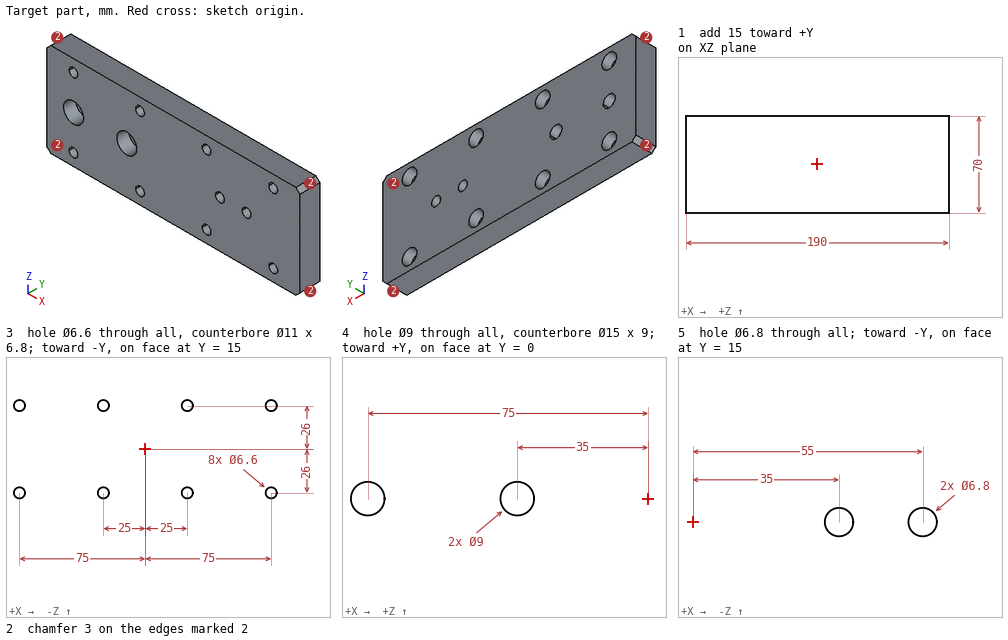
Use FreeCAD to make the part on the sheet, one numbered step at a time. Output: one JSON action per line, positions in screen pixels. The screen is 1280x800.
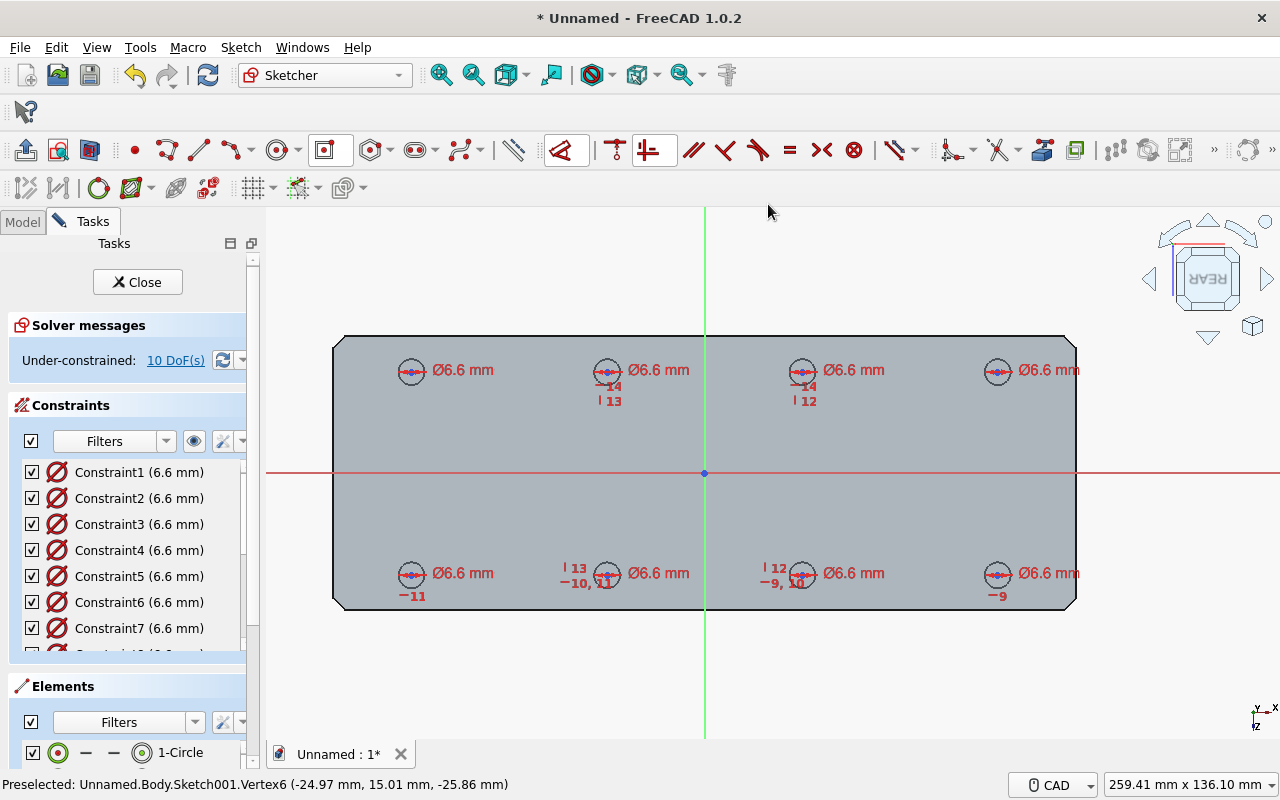
{"action": "left_click", "coordinate": [412, 575]}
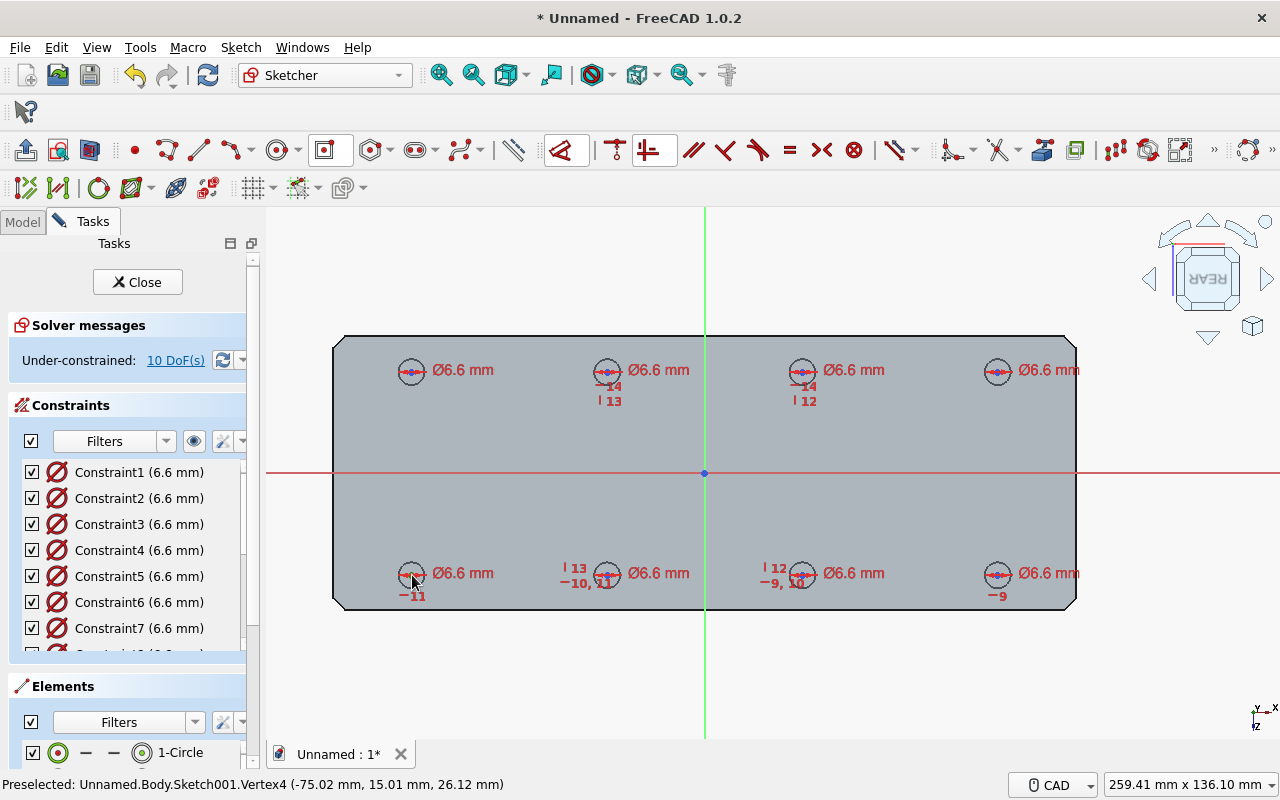
{"action": "left_click", "coordinate": [412, 372]}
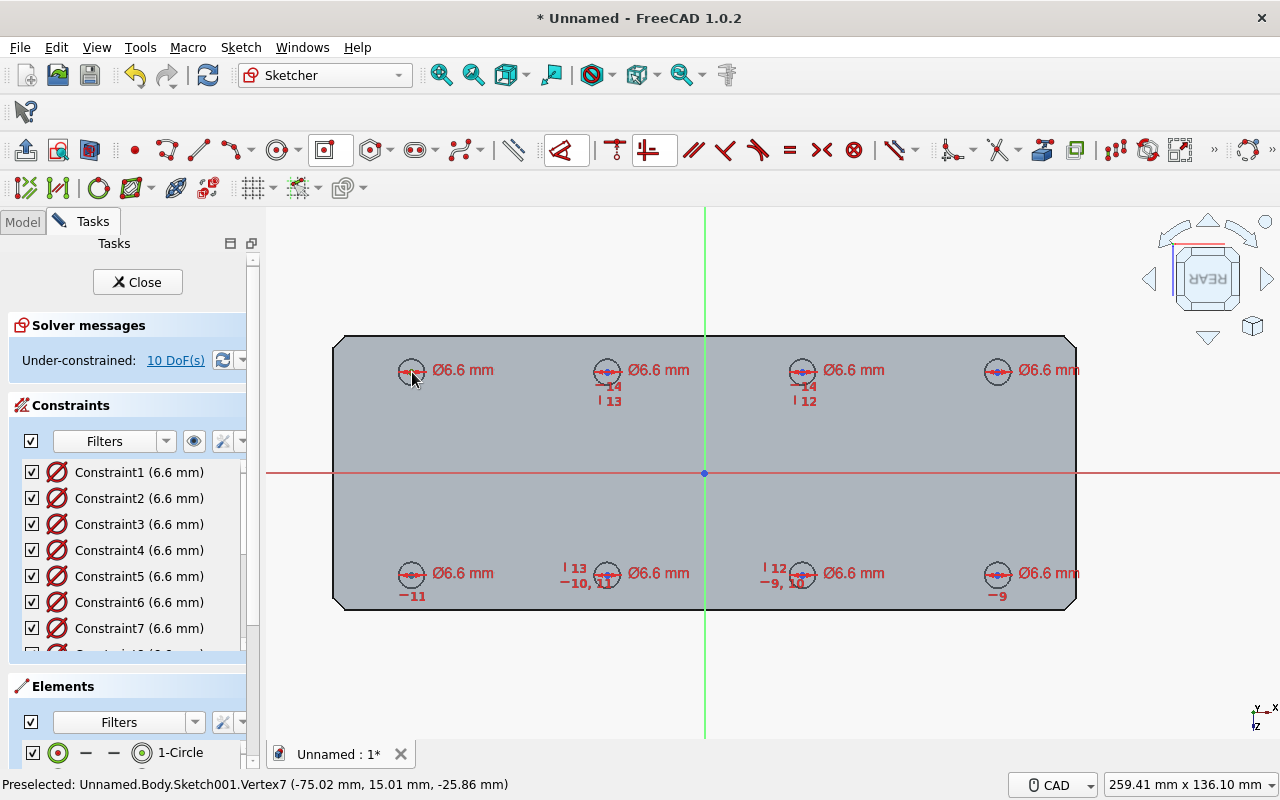
{"action": "key", "text": "v"}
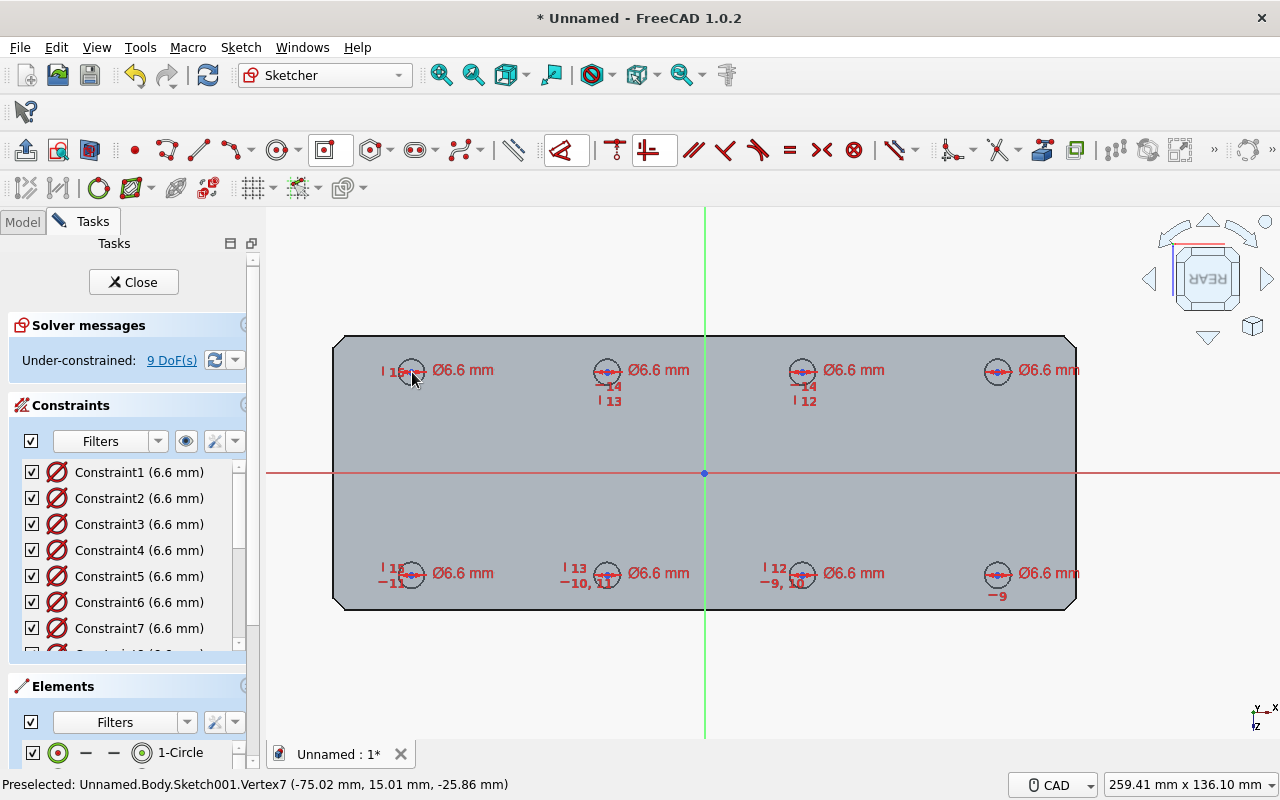
{"action": "left_click", "coordinate": [607, 372]}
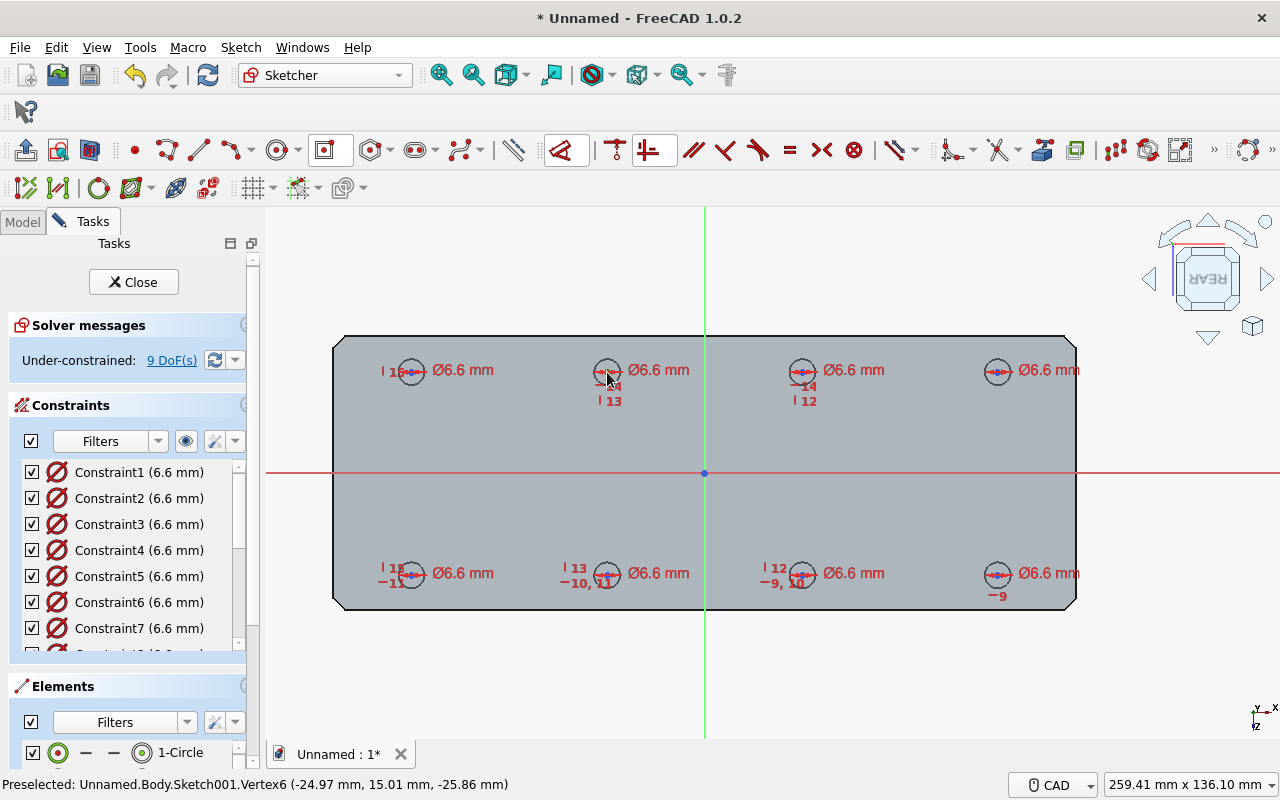
{"action": "left_click", "coordinate": [412, 372]}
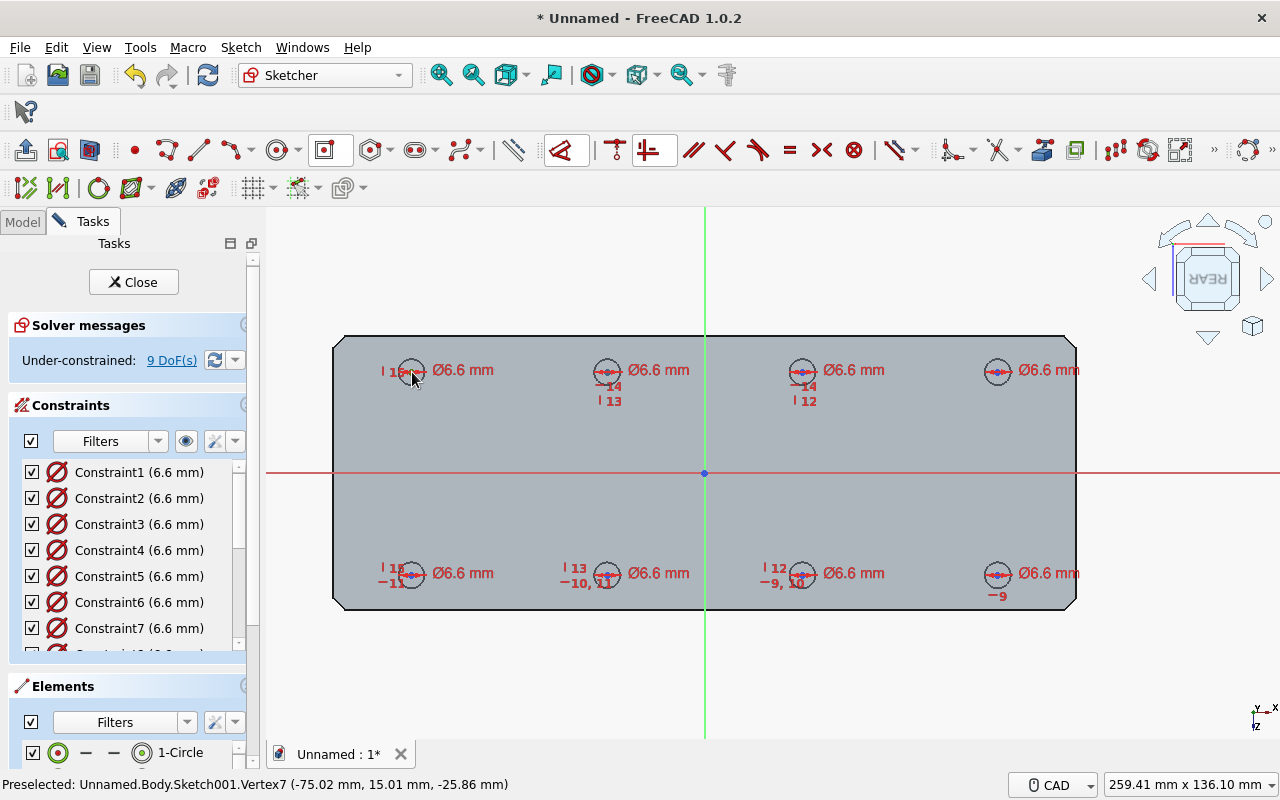
{"action": "key", "text": "h"}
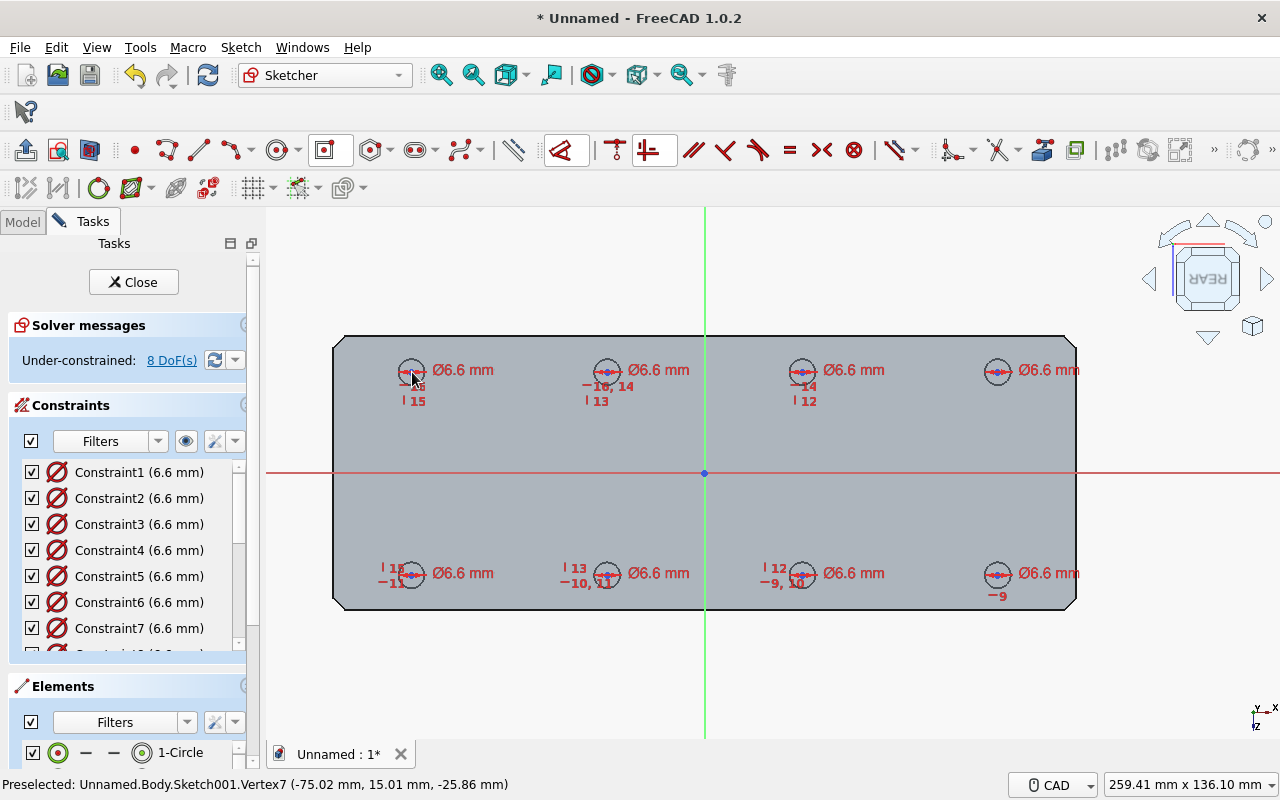
{"action": "left_click", "coordinate": [998, 575]}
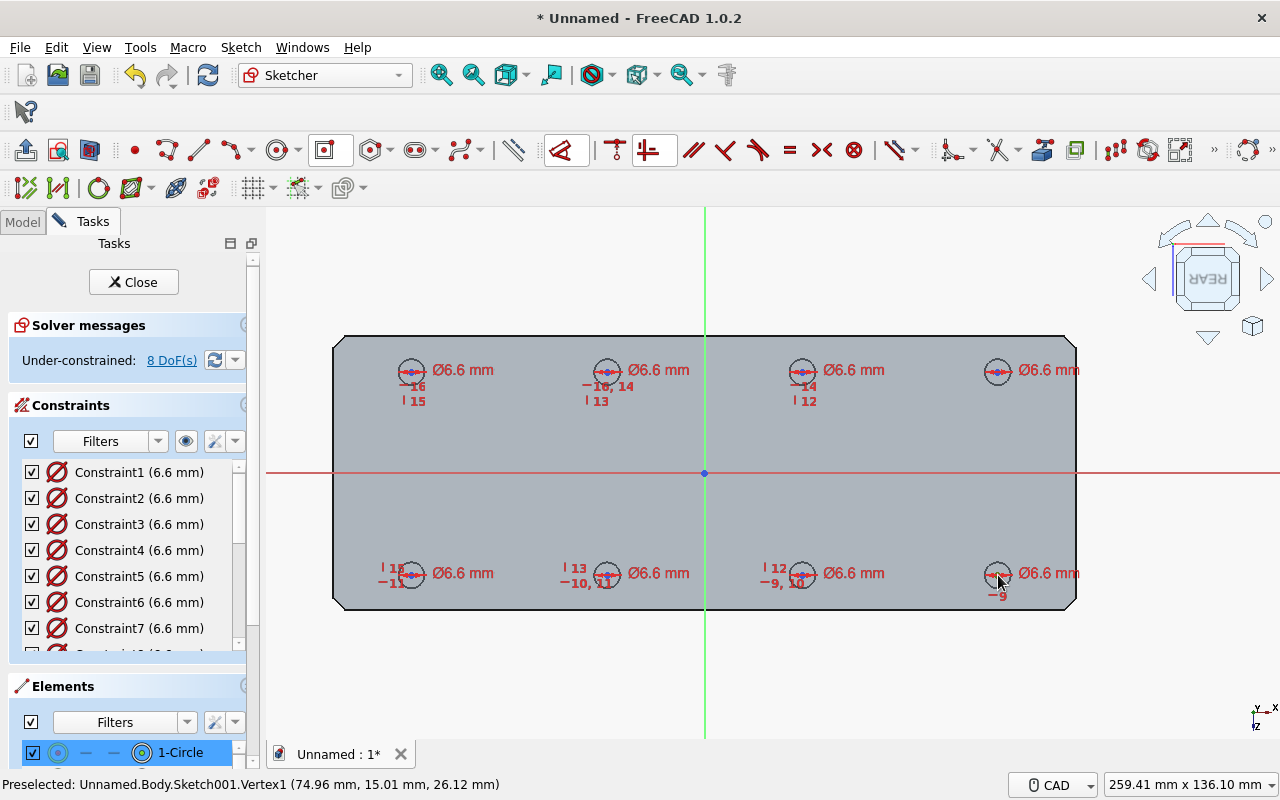
{"action": "left_click", "coordinate": [998, 372]}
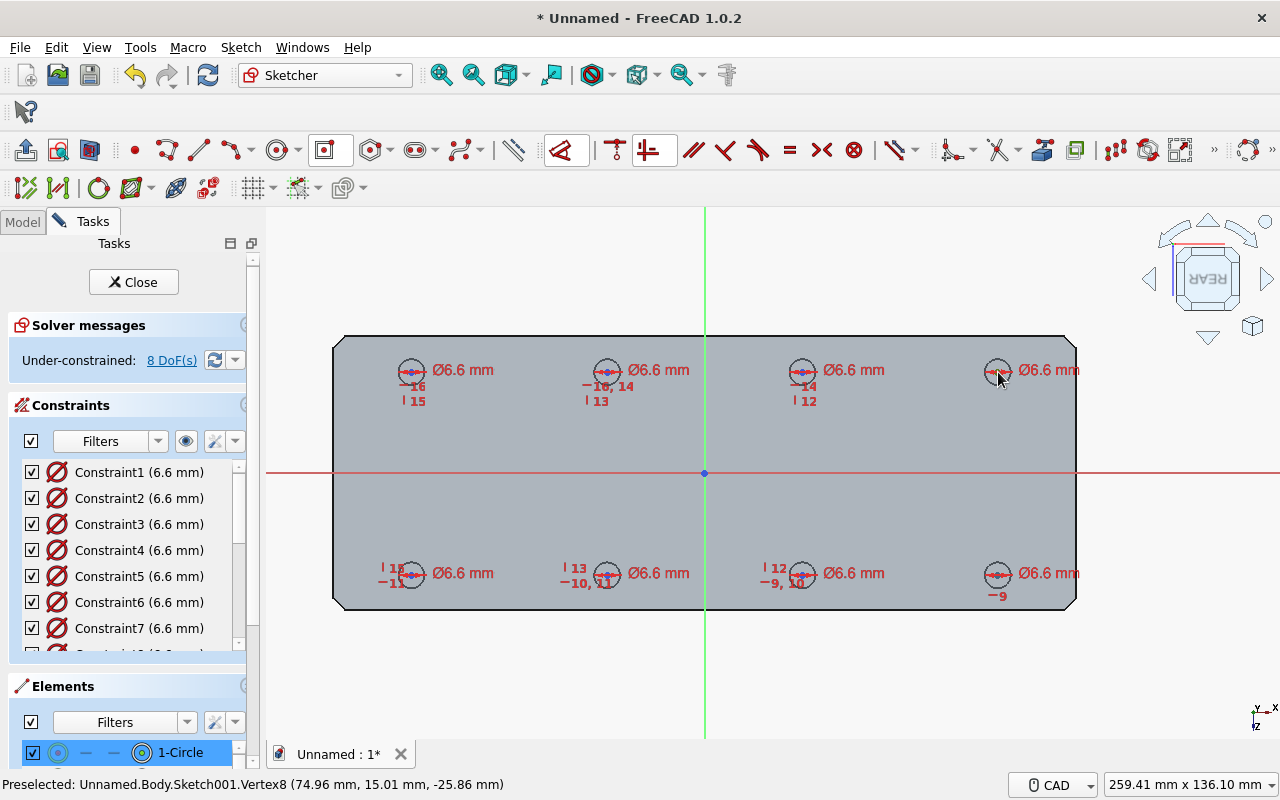
{"action": "key", "text": "v"}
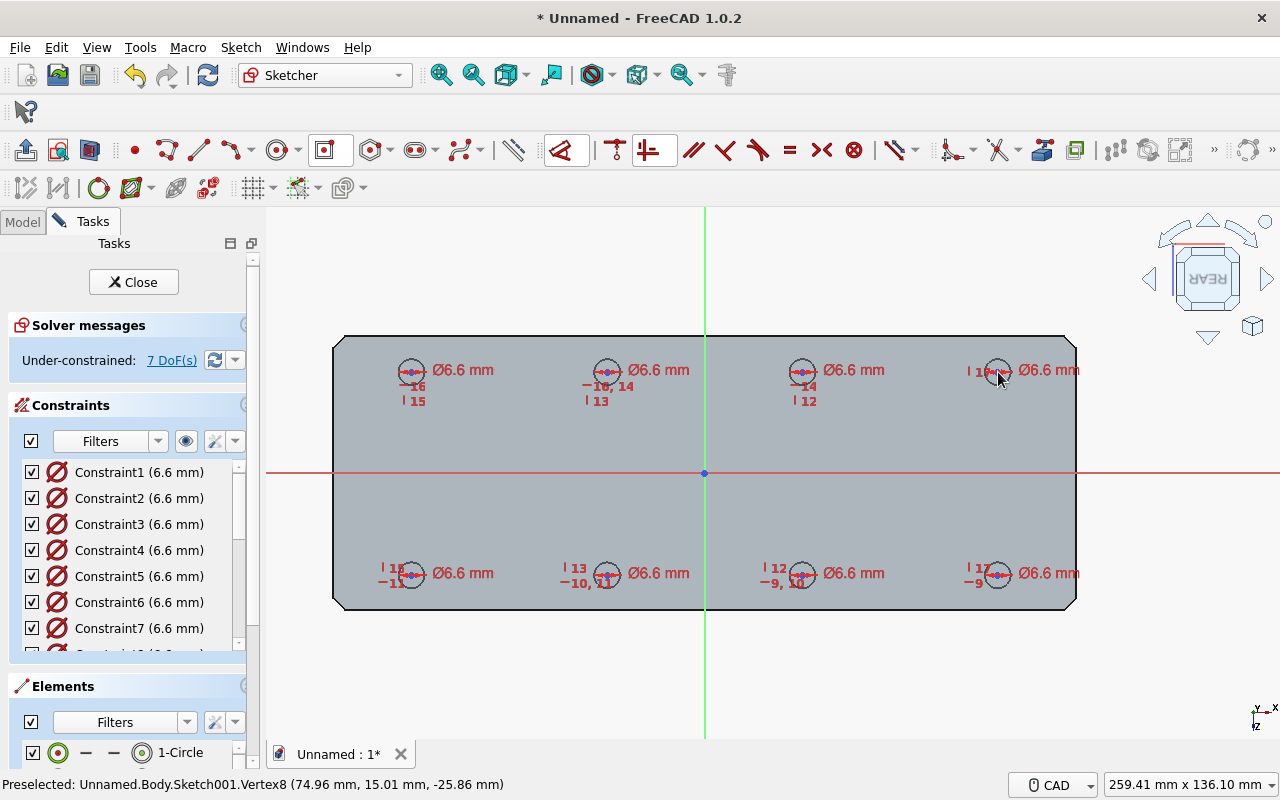
{"action": "left_click", "coordinate": [802, 372]}